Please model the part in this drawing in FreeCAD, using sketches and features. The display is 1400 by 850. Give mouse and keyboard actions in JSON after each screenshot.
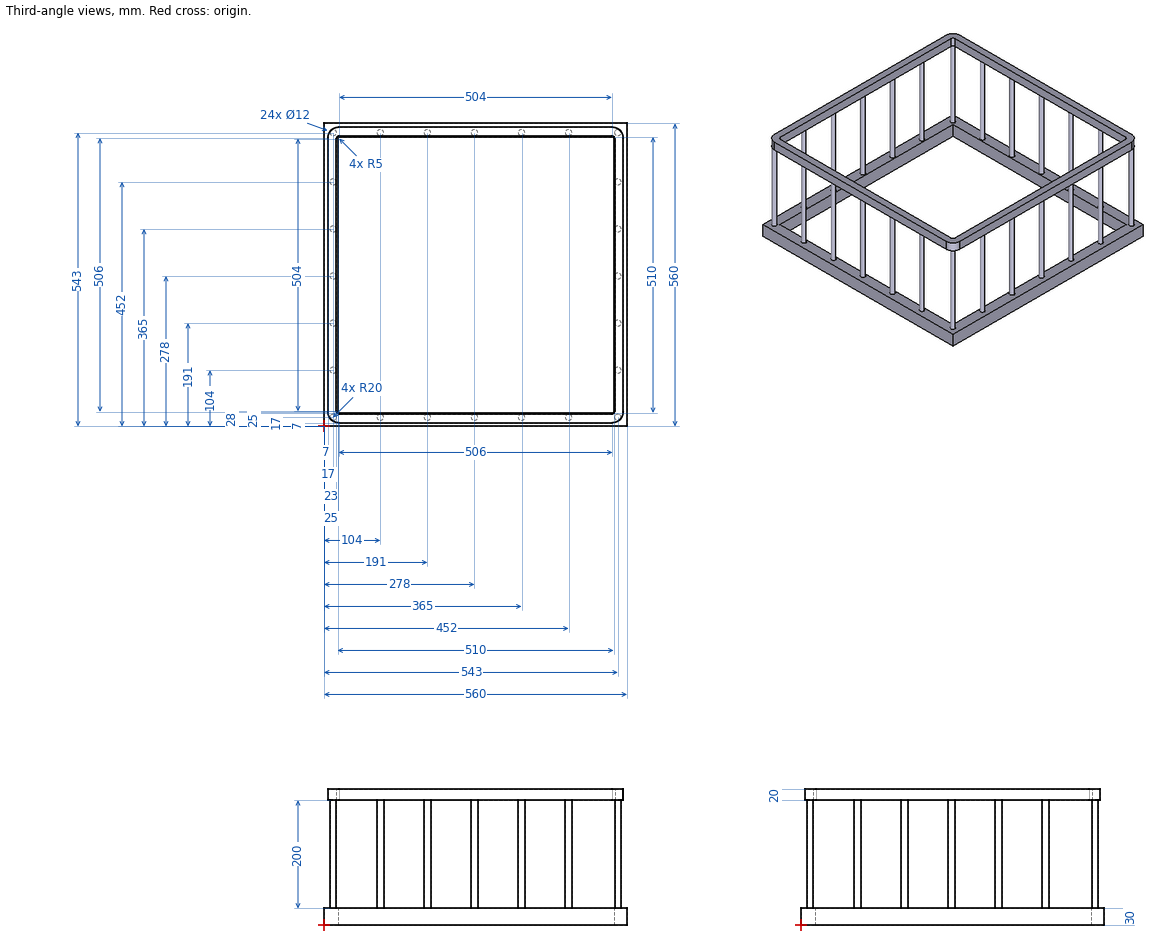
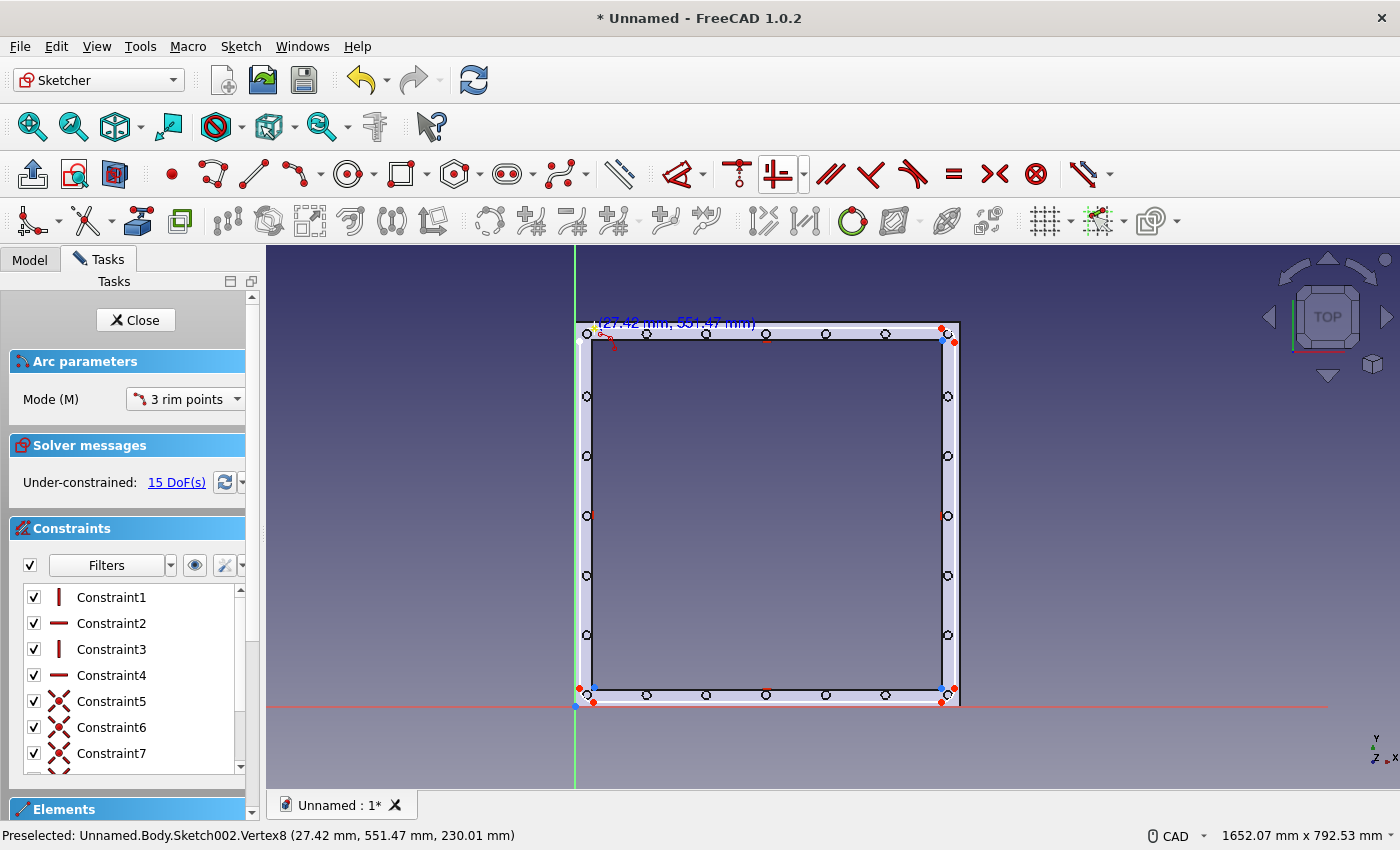
{"action": "scroll", "coordinate": [580, 341], "scroll_direction": "up", "scroll_amount": 6}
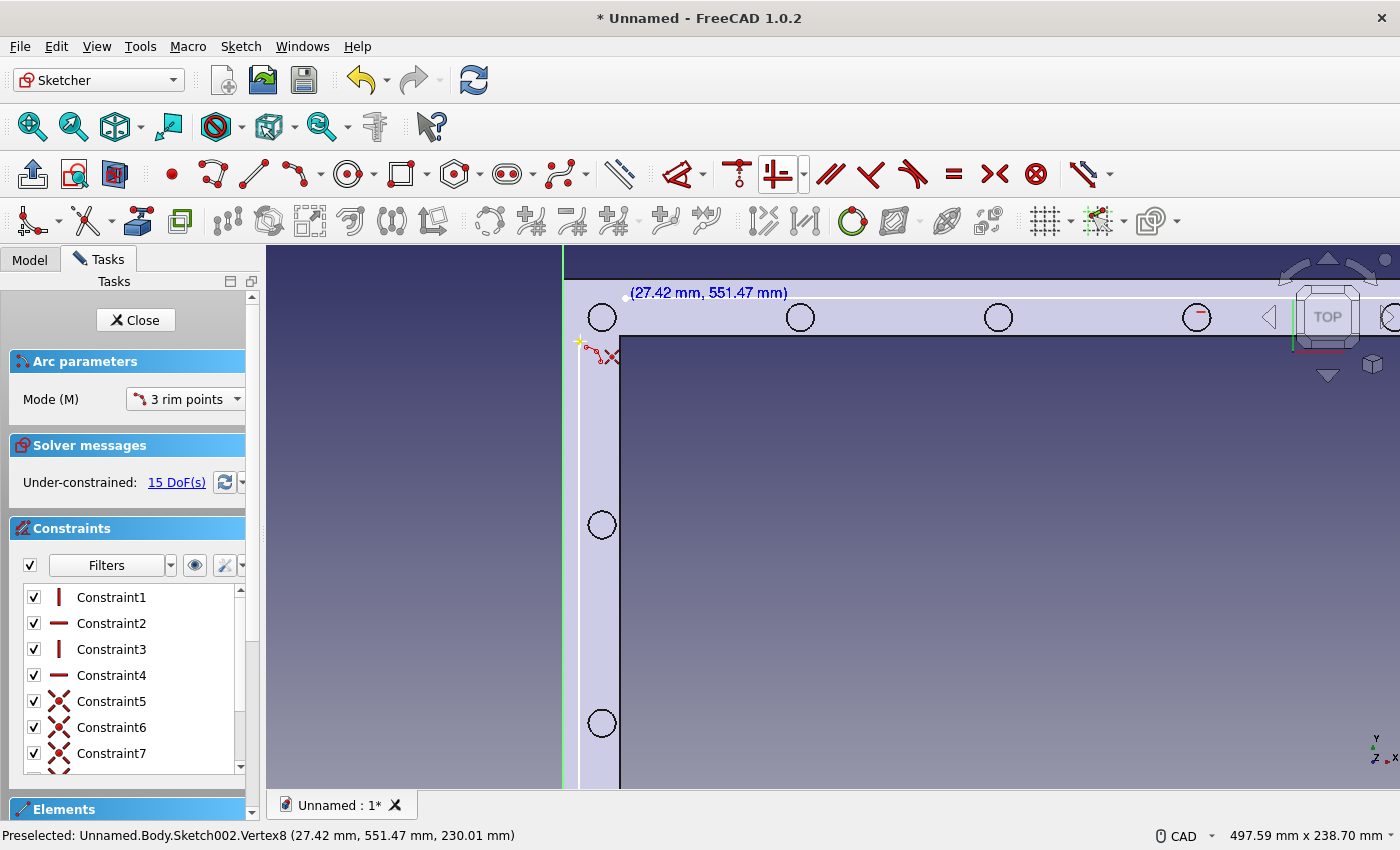
{"action": "left_click", "coordinate": [579, 342]}
{"action": "left_click", "coordinate": [593, 308]}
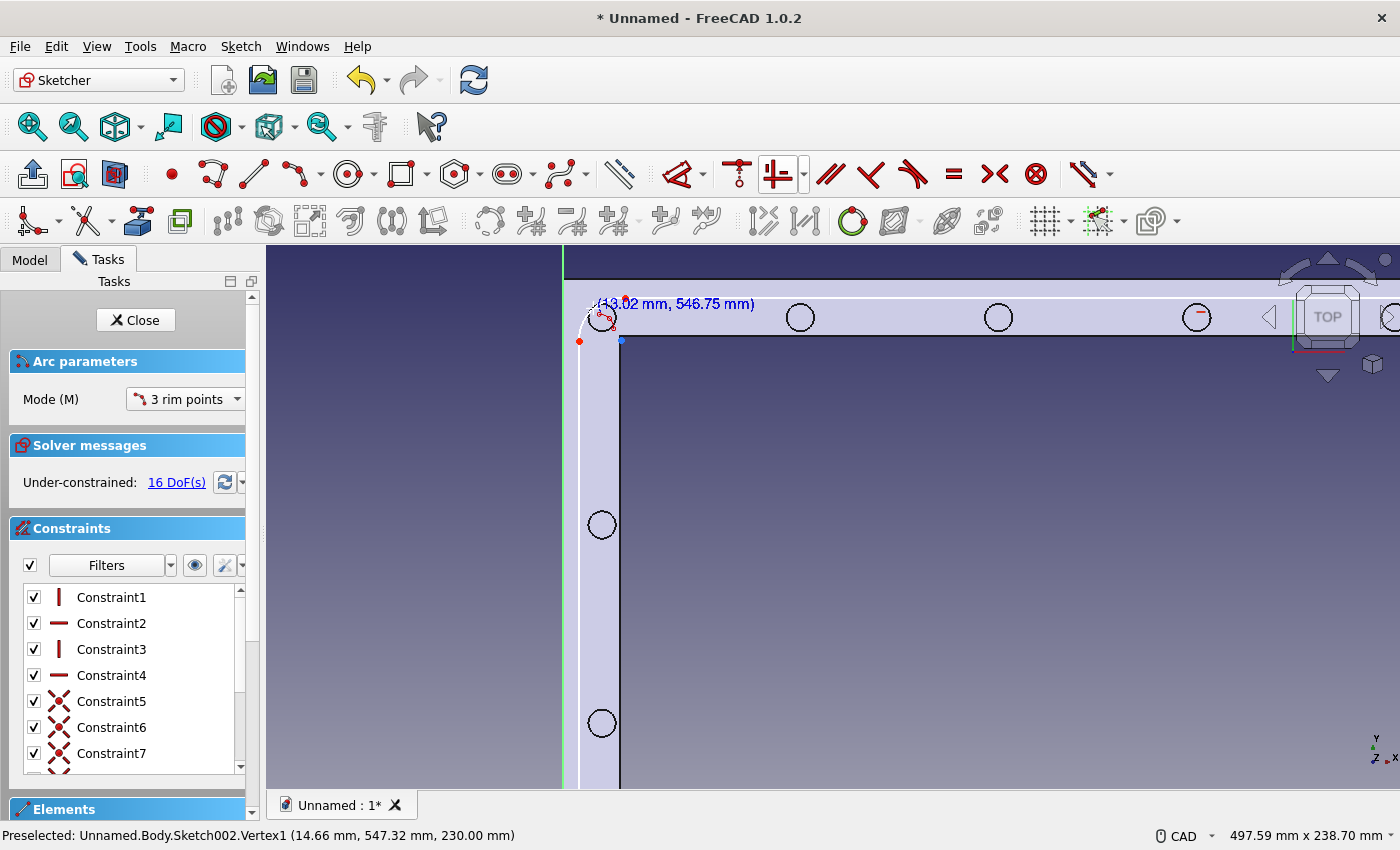
{"action": "left_click", "coordinate": [254, 174]}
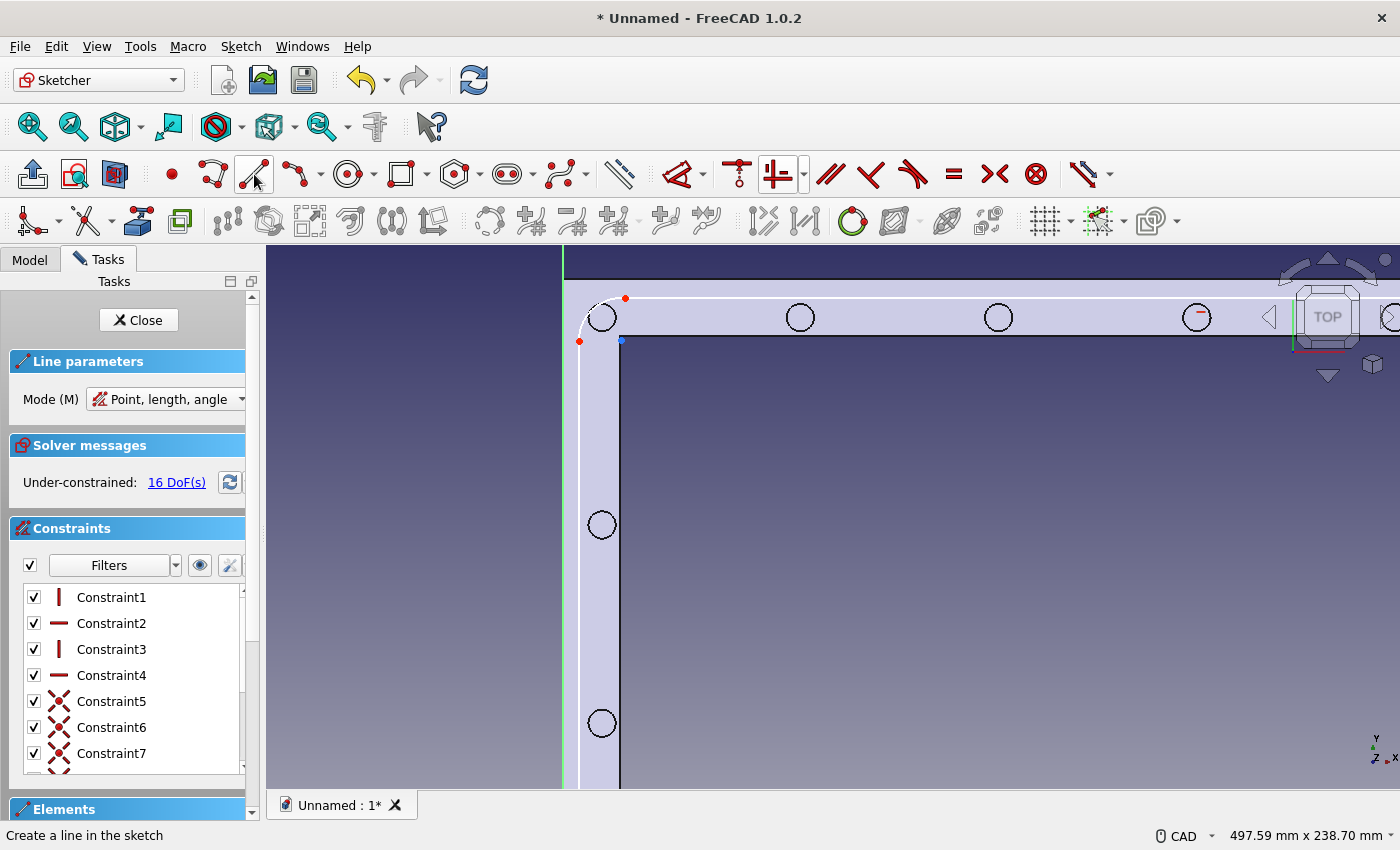
{"action": "scroll", "coordinate": [580, 341], "scroll_direction": "down", "scroll_amount": 6}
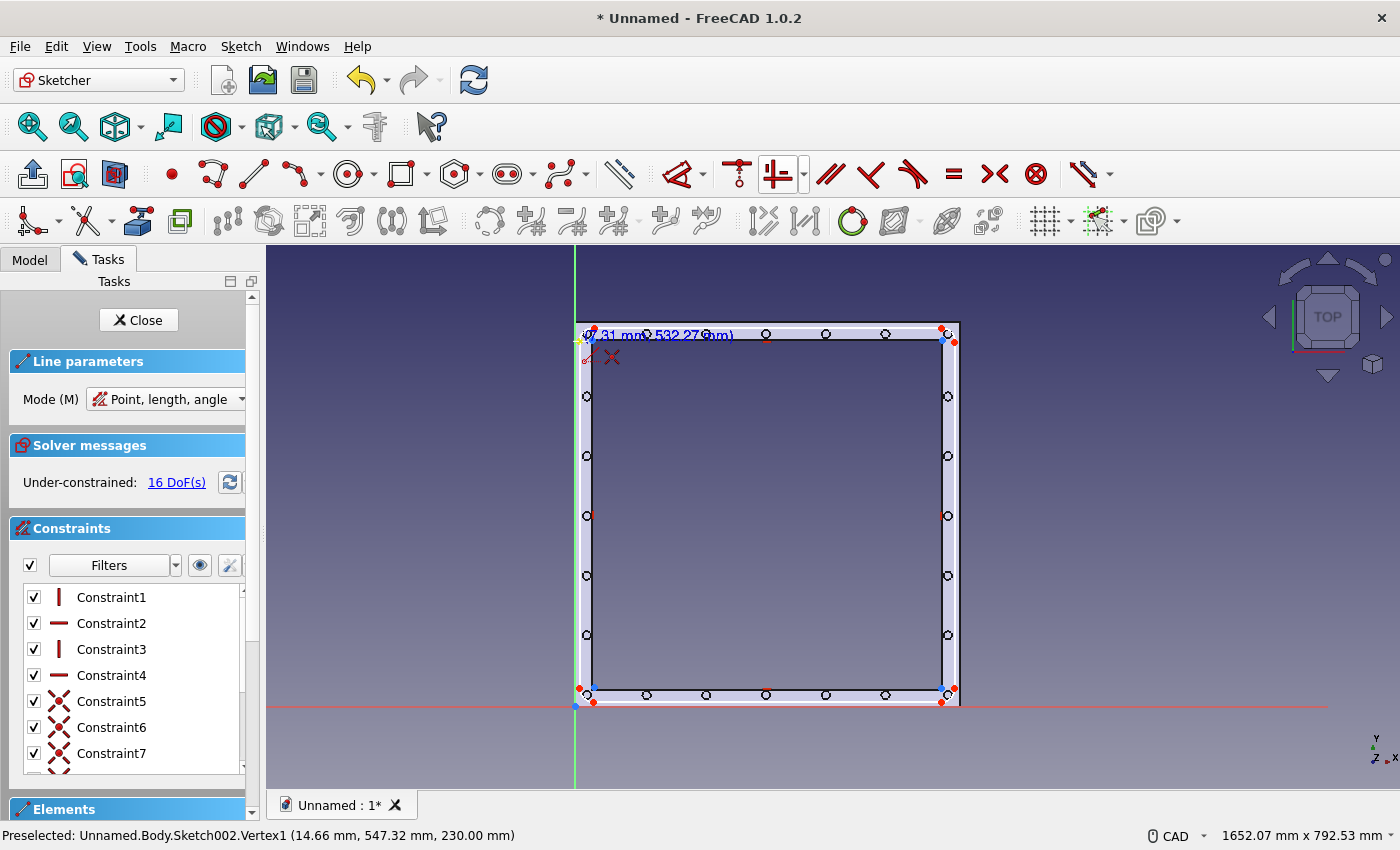
{"action": "scroll", "coordinate": [591, 688], "scroll_direction": "up", "scroll_amount": 9}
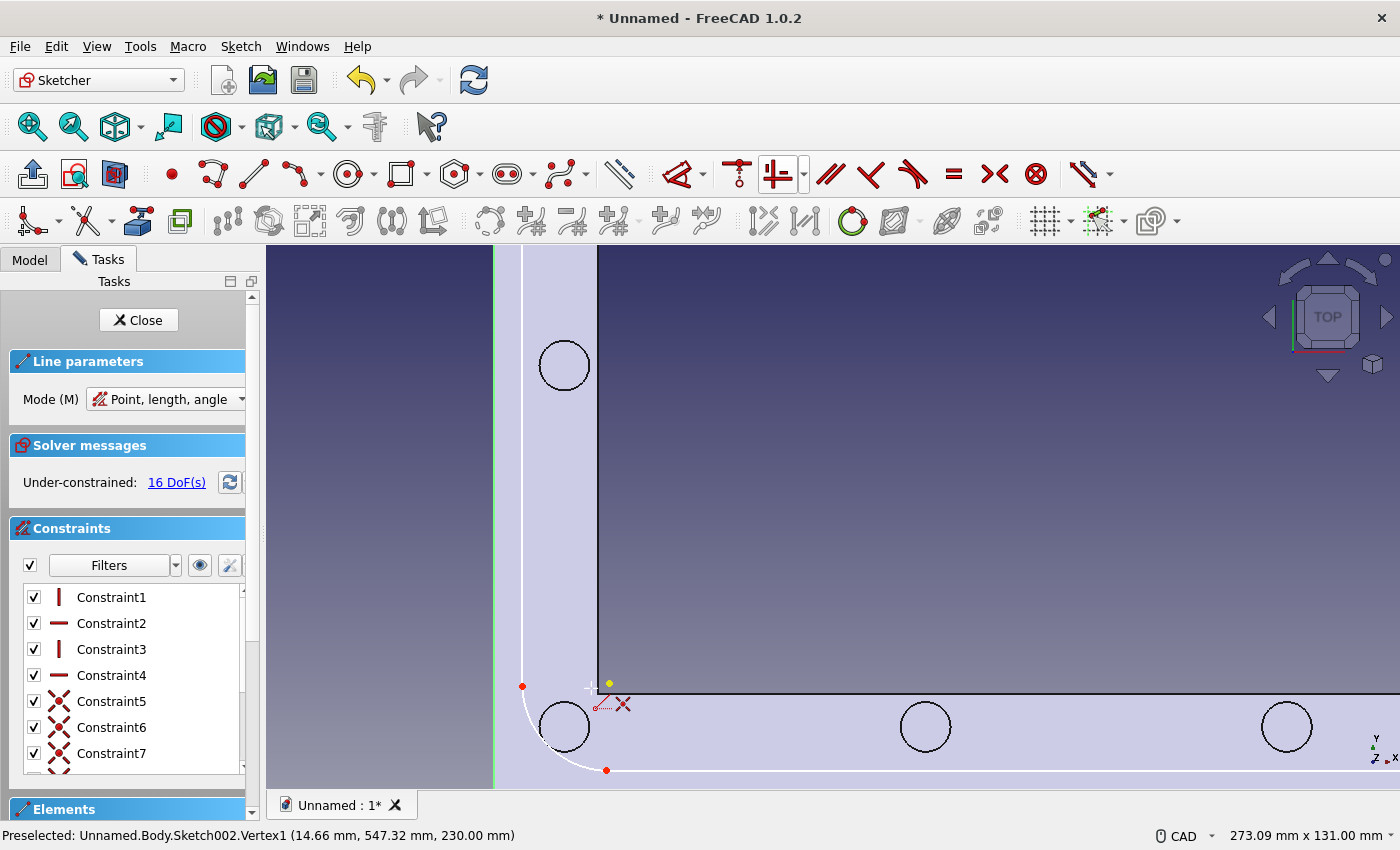
{"action": "left_click", "coordinate": [589, 681]}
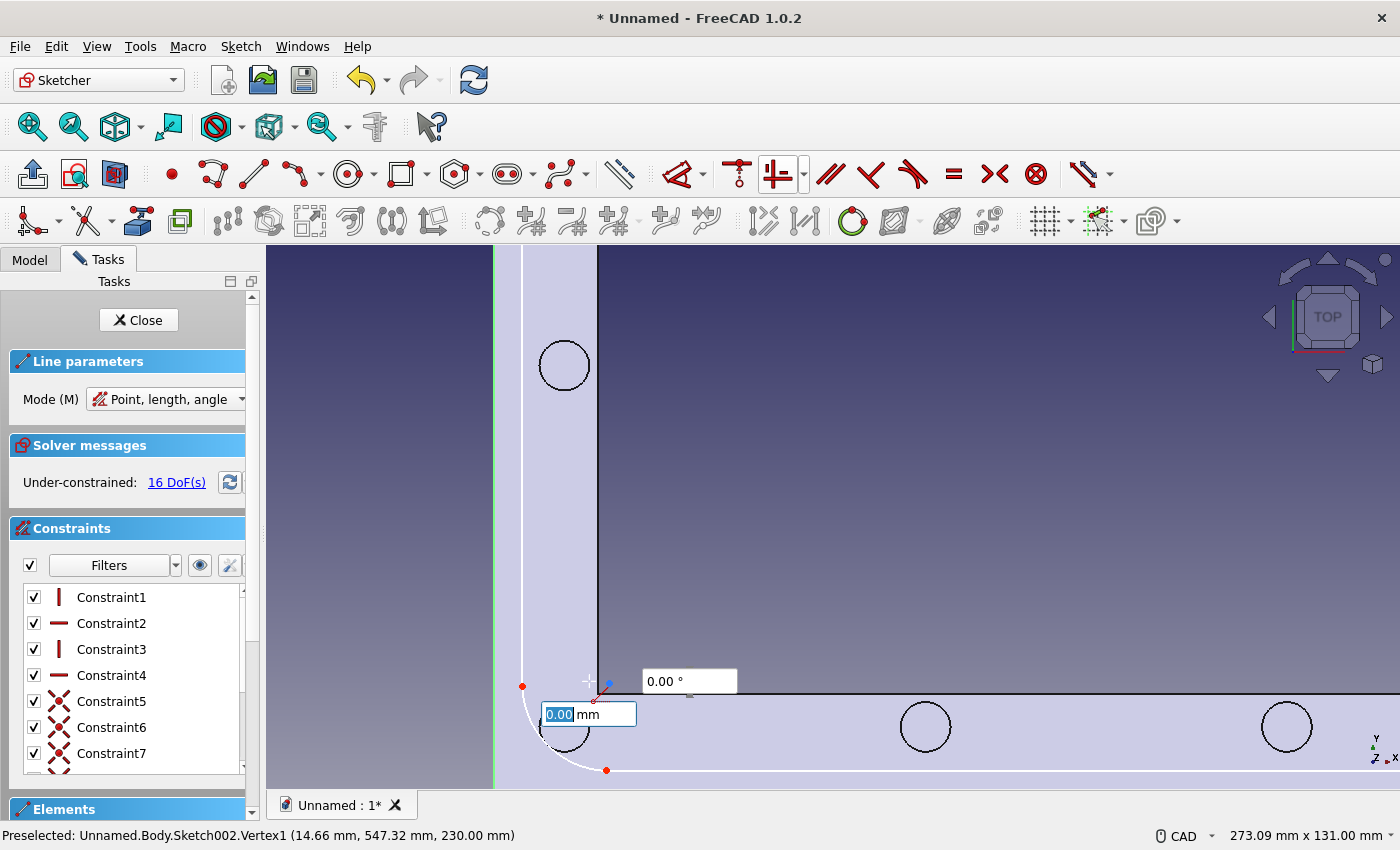
{"action": "scroll", "coordinate": [591, 689], "scroll_direction": "down", "scroll_amount": 9}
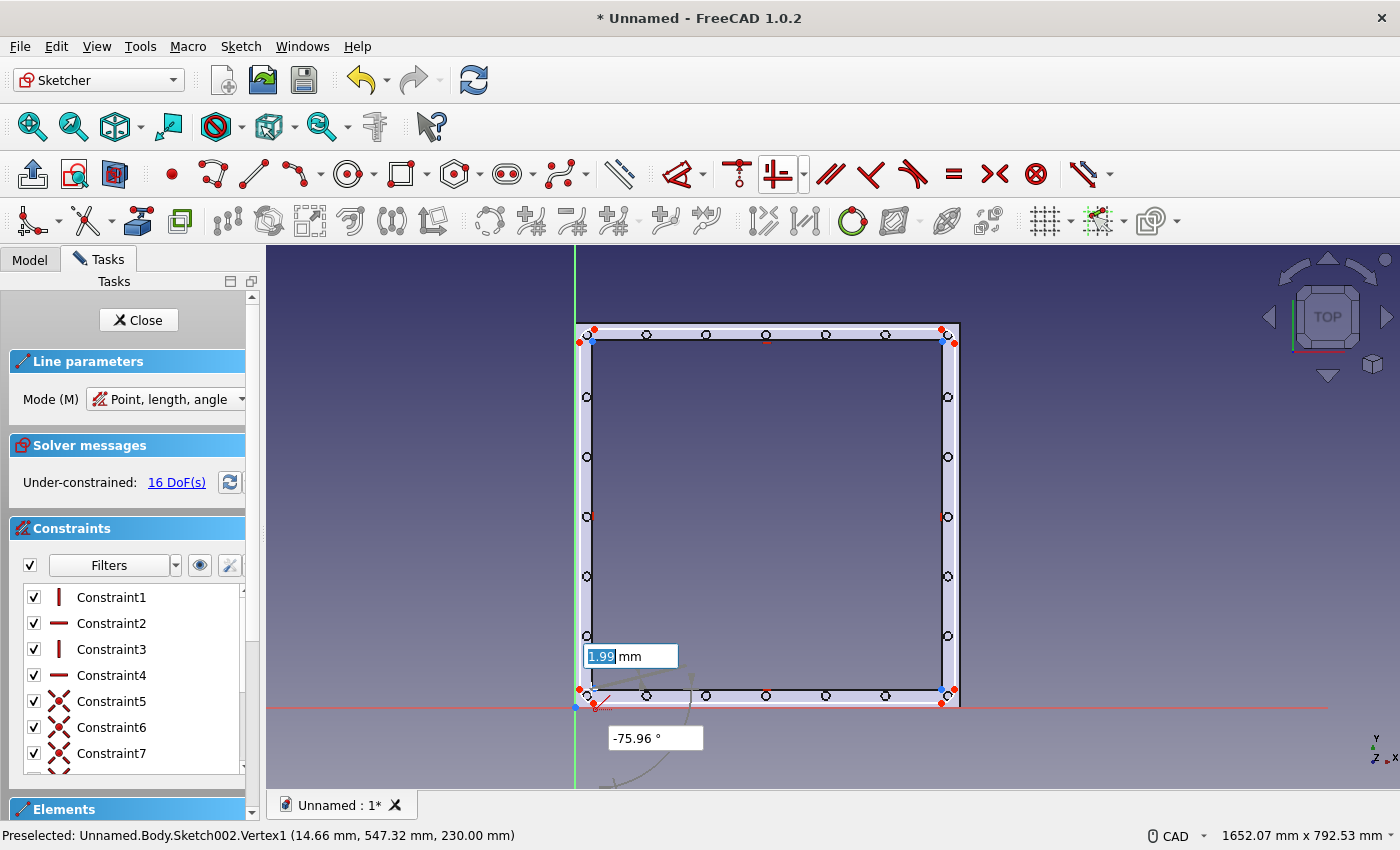
{"action": "scroll", "coordinate": [591, 342], "scroll_direction": "up", "scroll_amount": 9}